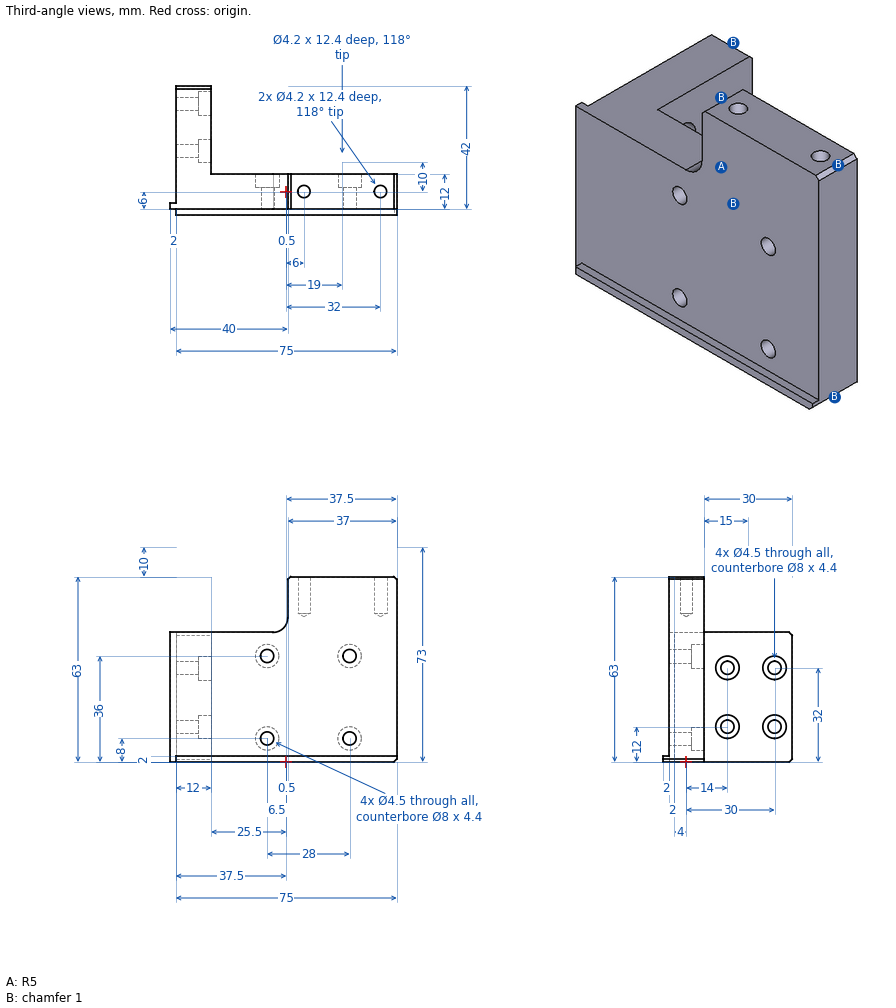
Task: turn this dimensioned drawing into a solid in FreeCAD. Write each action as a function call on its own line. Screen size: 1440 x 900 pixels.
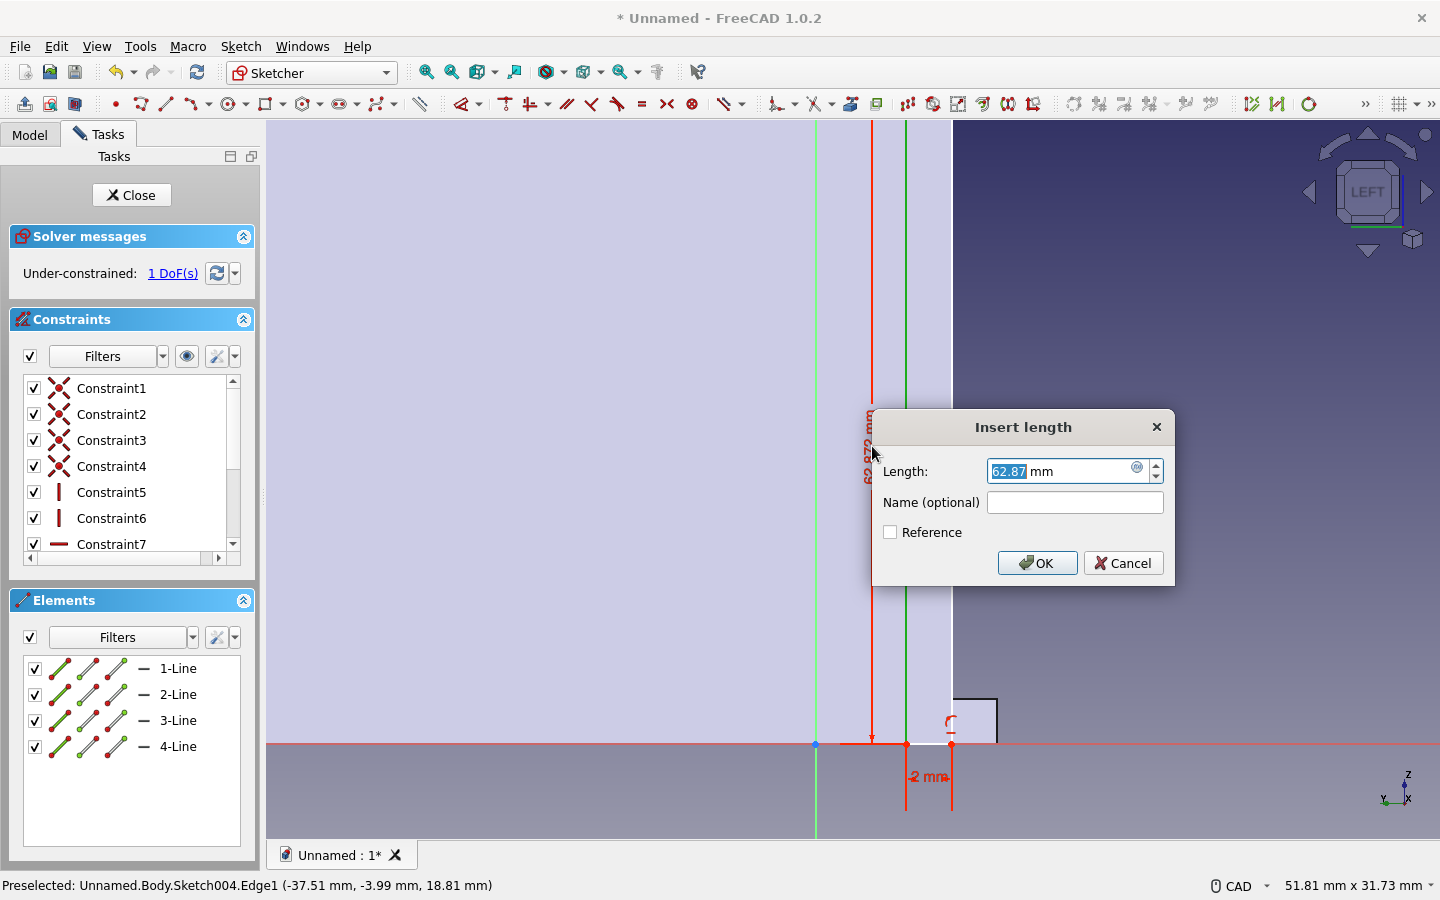
text(63)
key(Return)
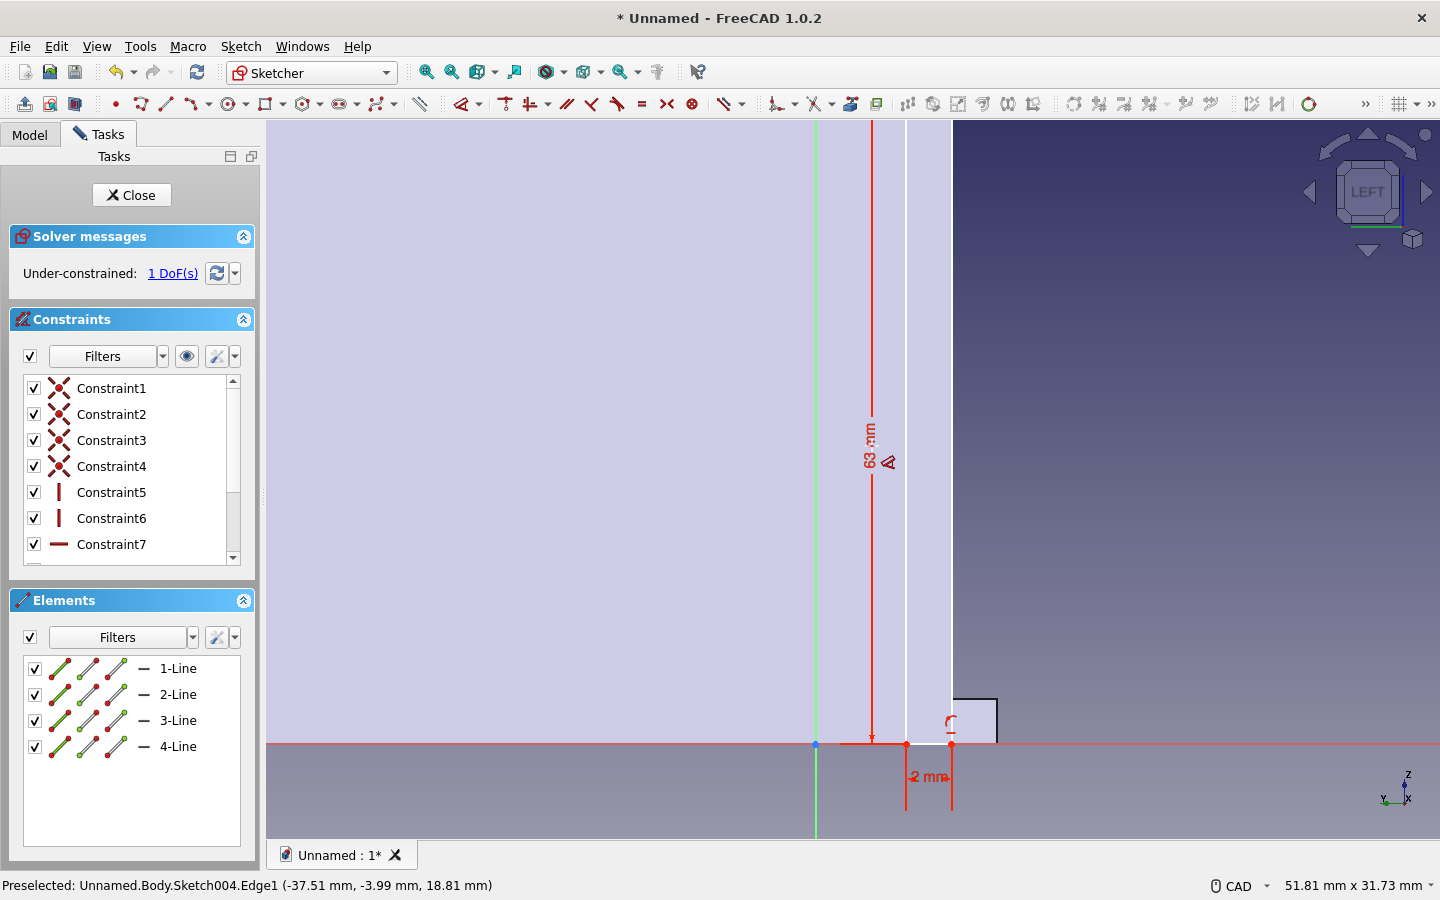
scroll(742, 673, down, 6)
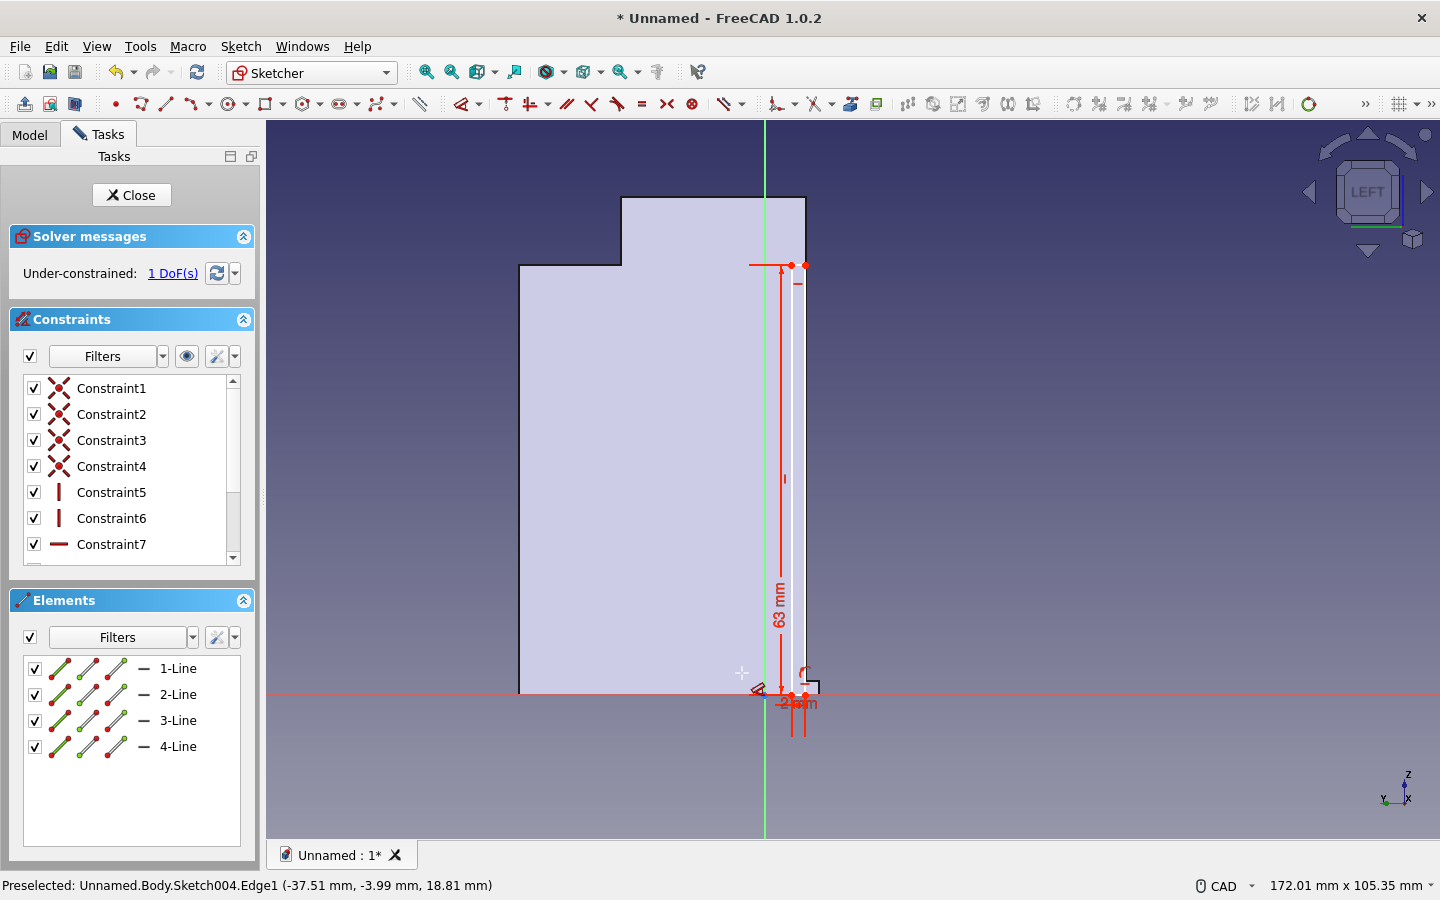
scroll(792, 265, up, 2)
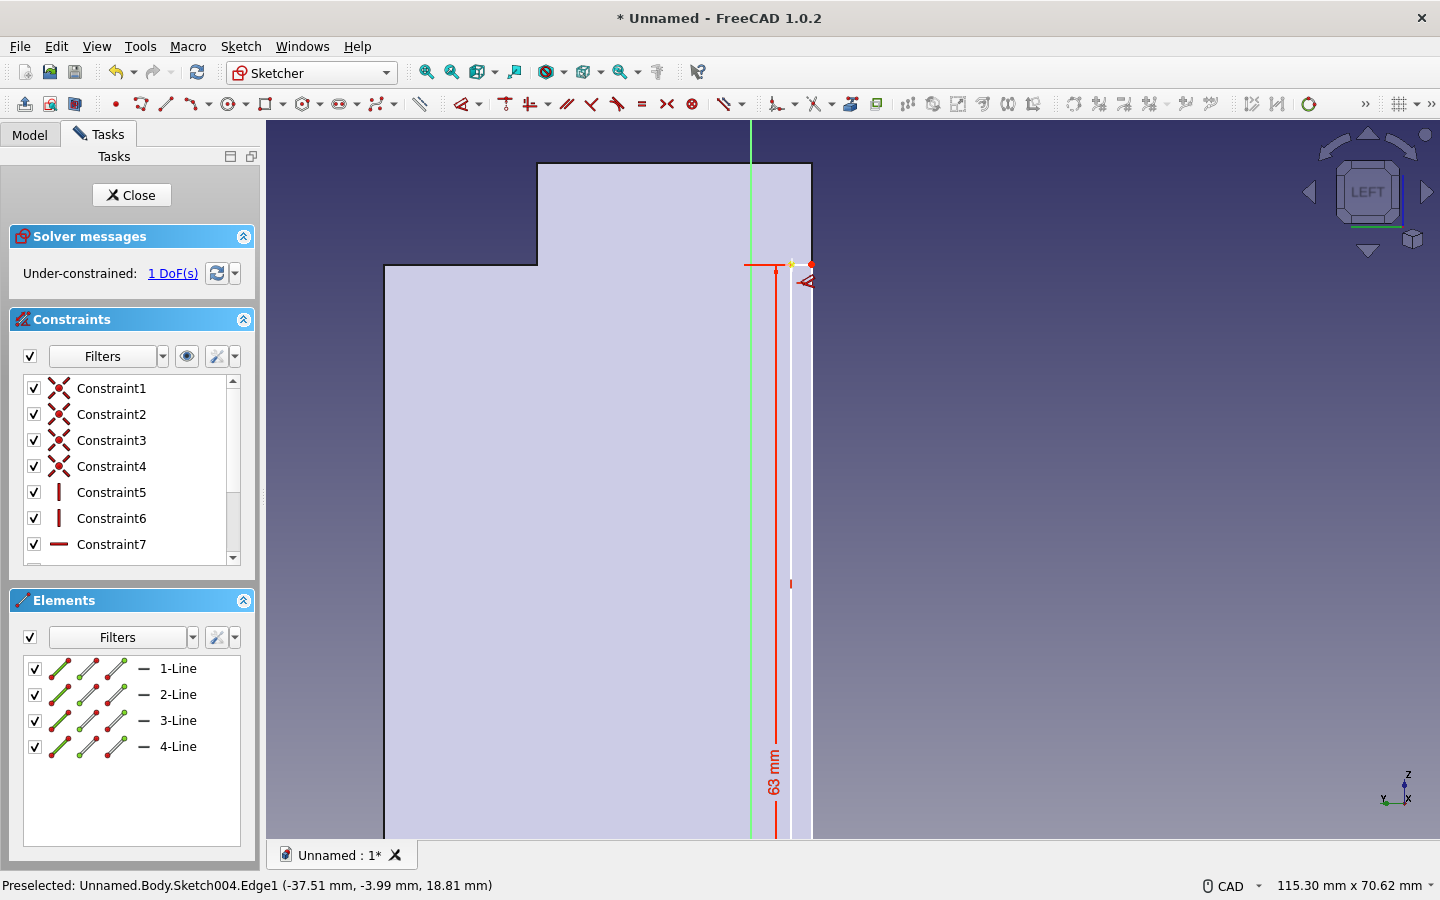
click(792, 265)
click(771, 231)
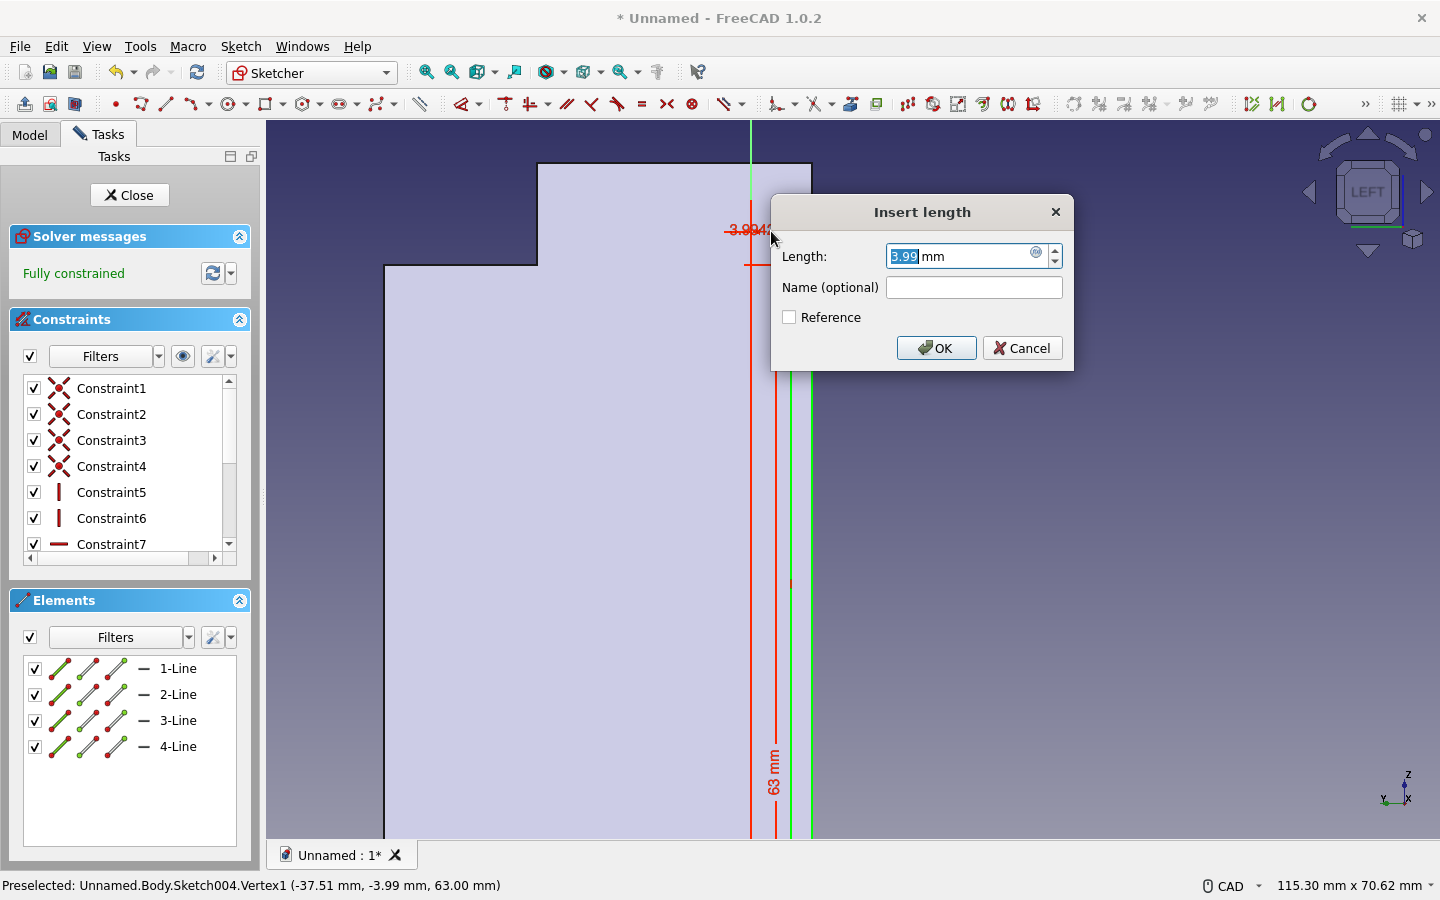
text(4)
key(Return)
key(Escape)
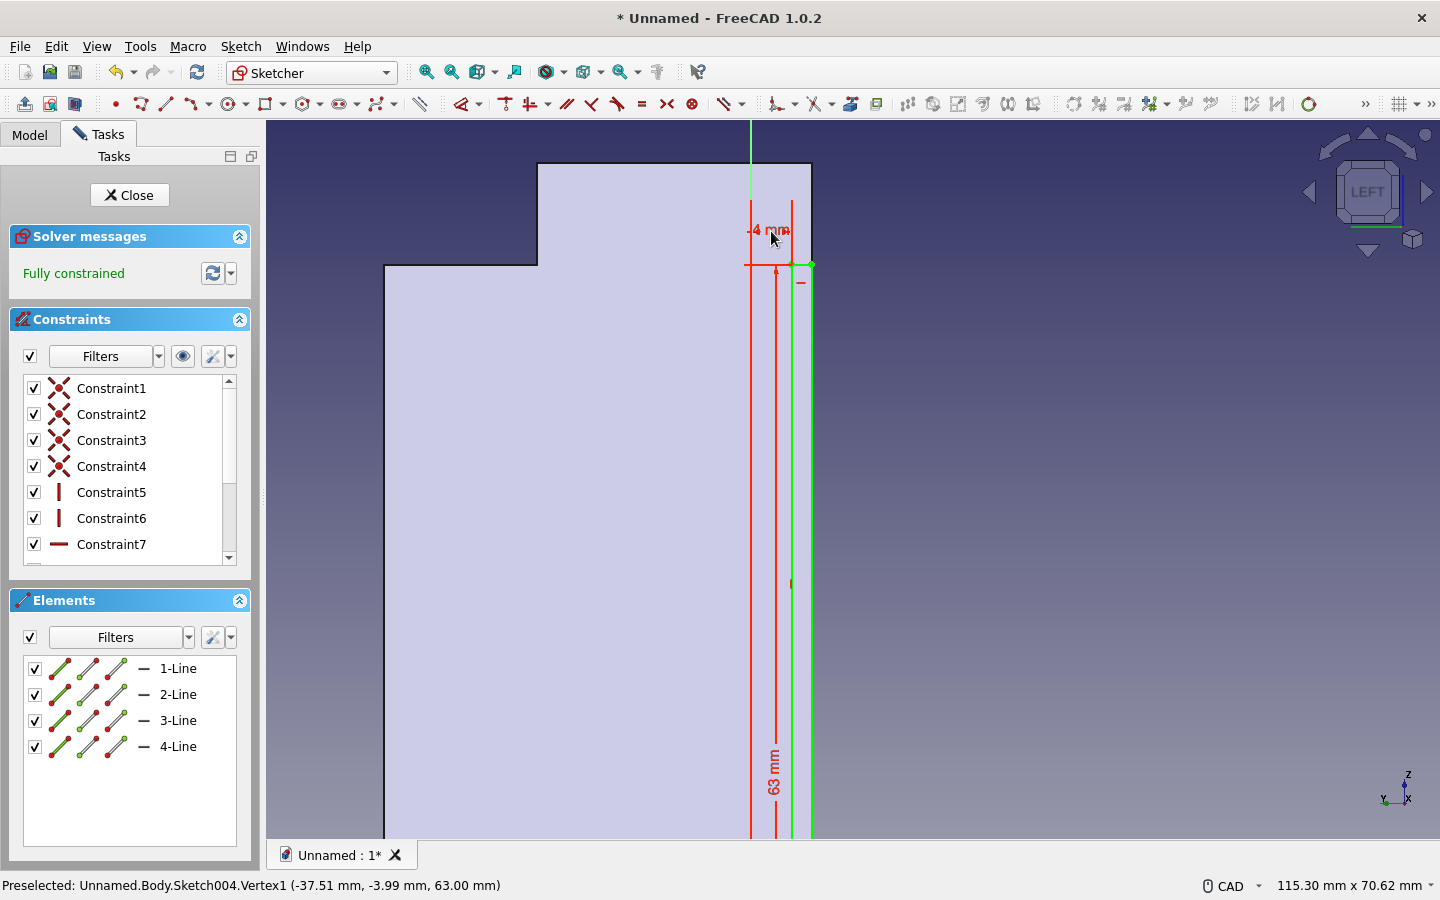
click(130, 195)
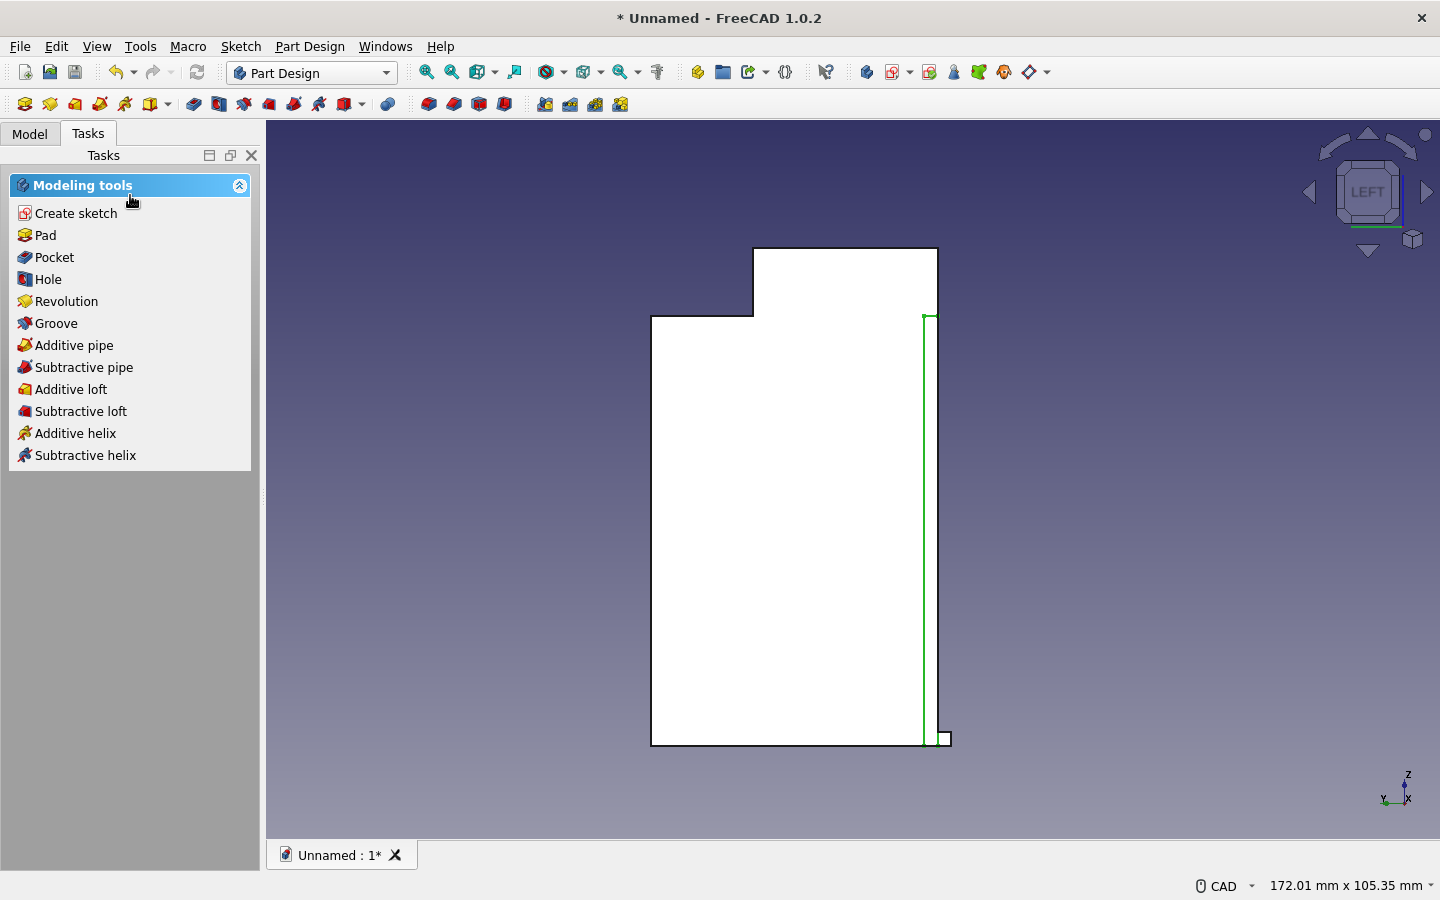
click(25, 104)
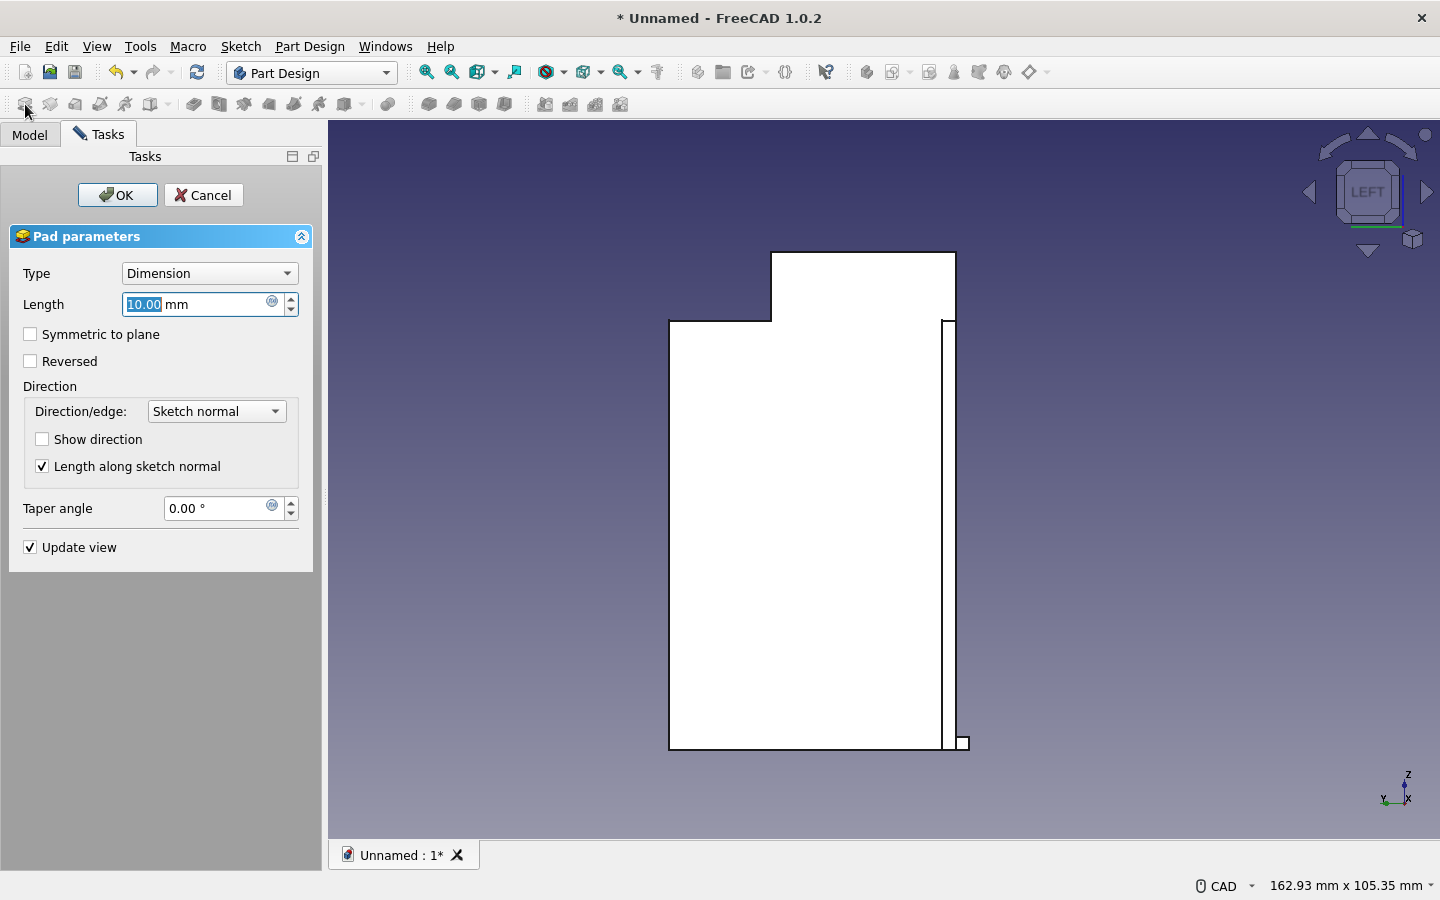
text(2)
key(Tab)